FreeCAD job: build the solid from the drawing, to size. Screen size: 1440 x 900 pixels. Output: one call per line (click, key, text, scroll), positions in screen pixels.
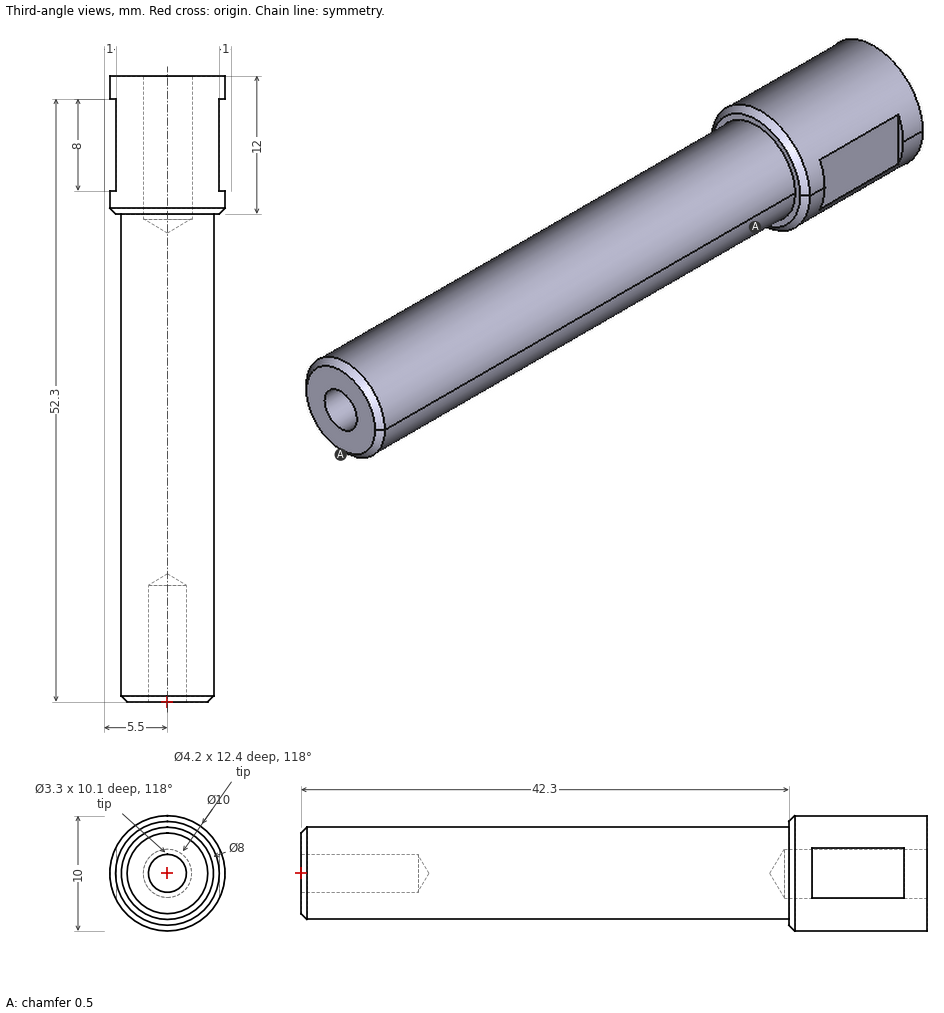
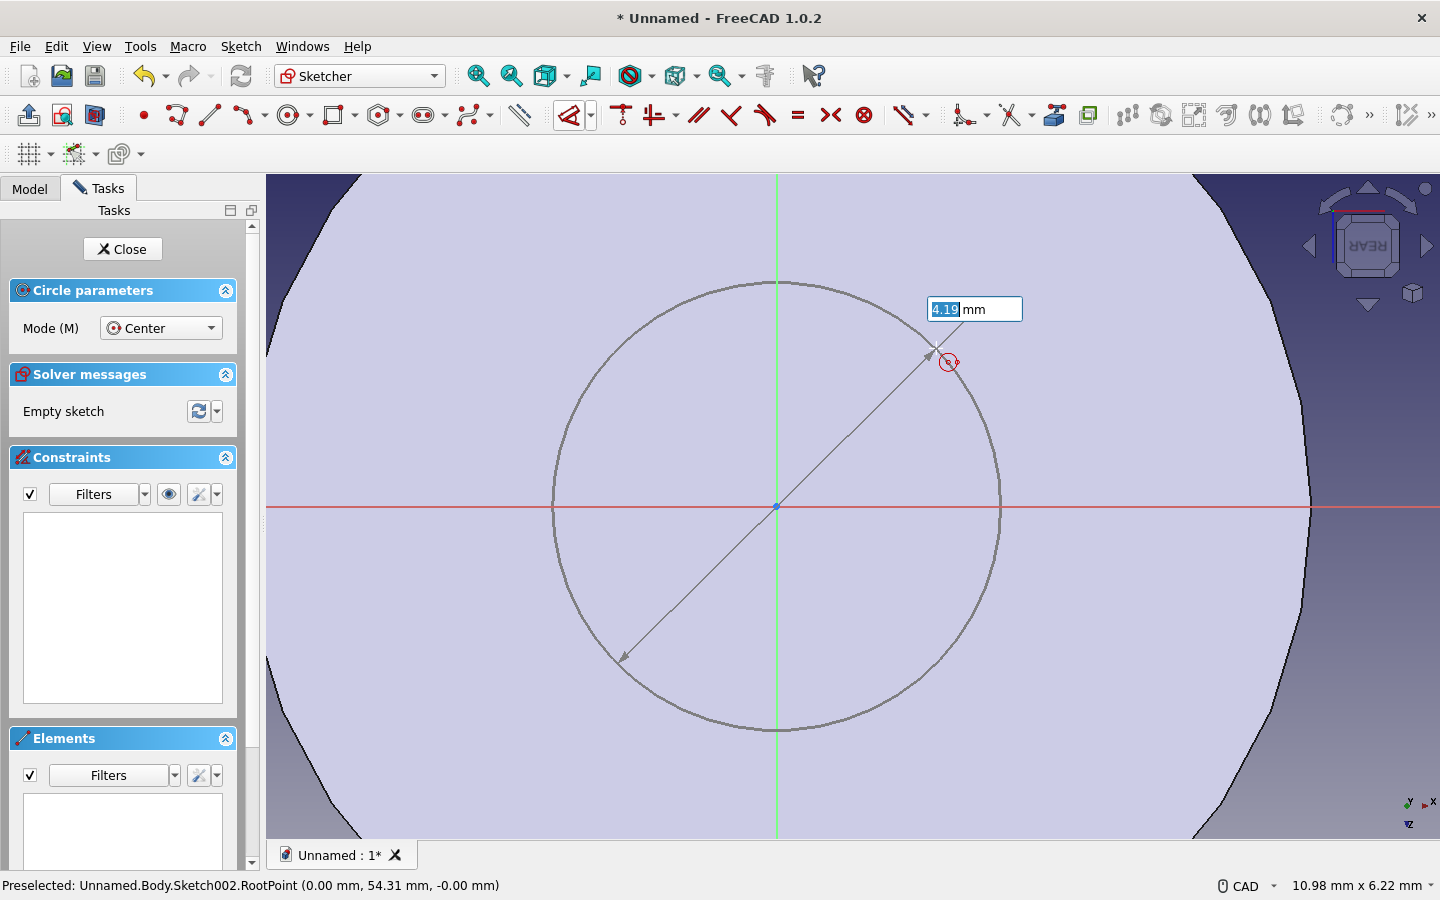
text(4.2)
key(Return)
key(Escape)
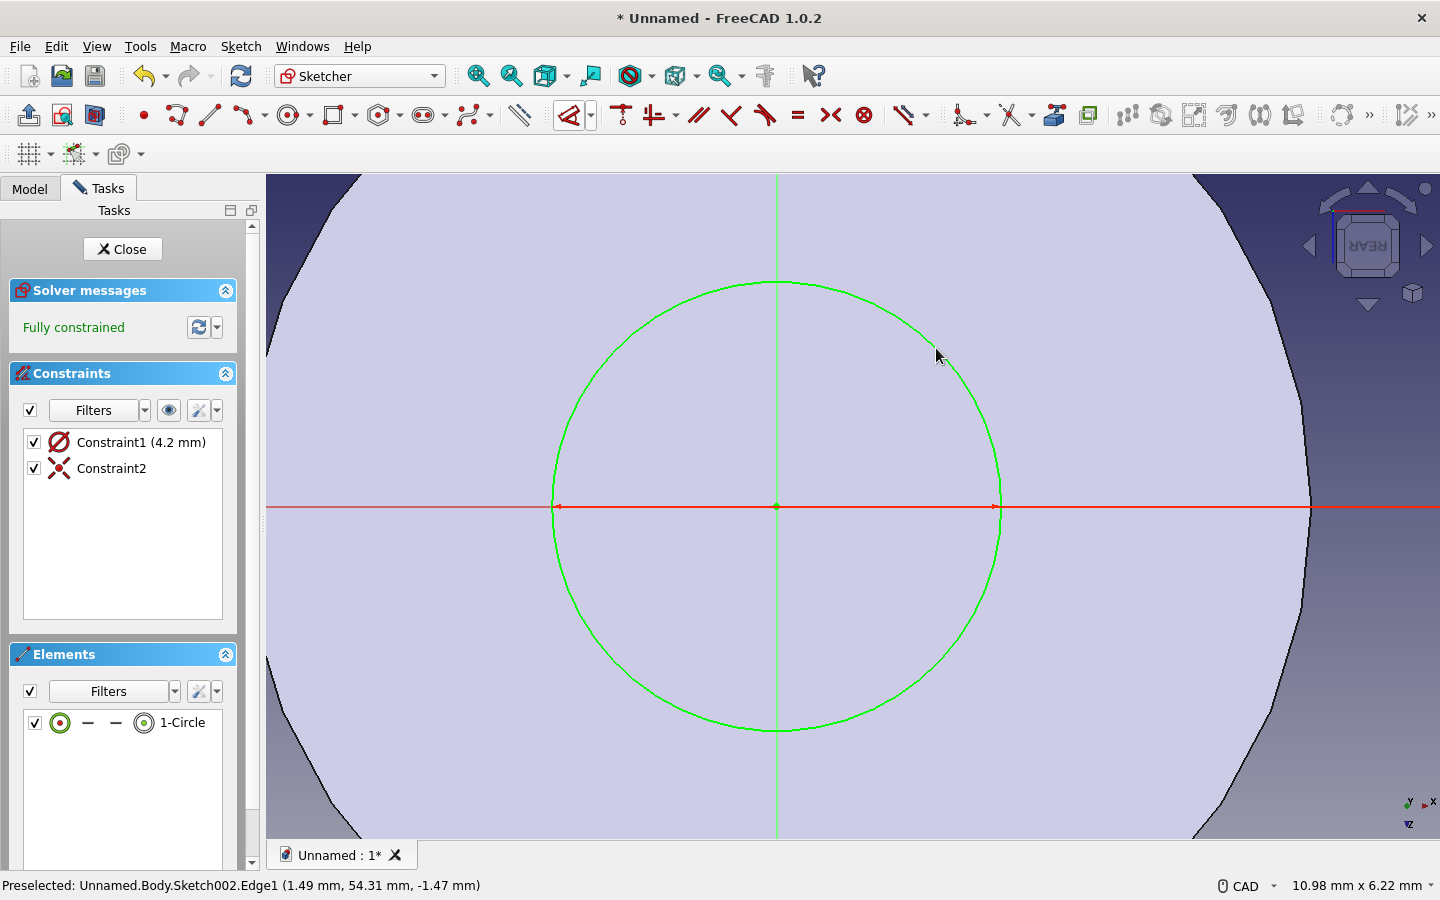
click(123, 249)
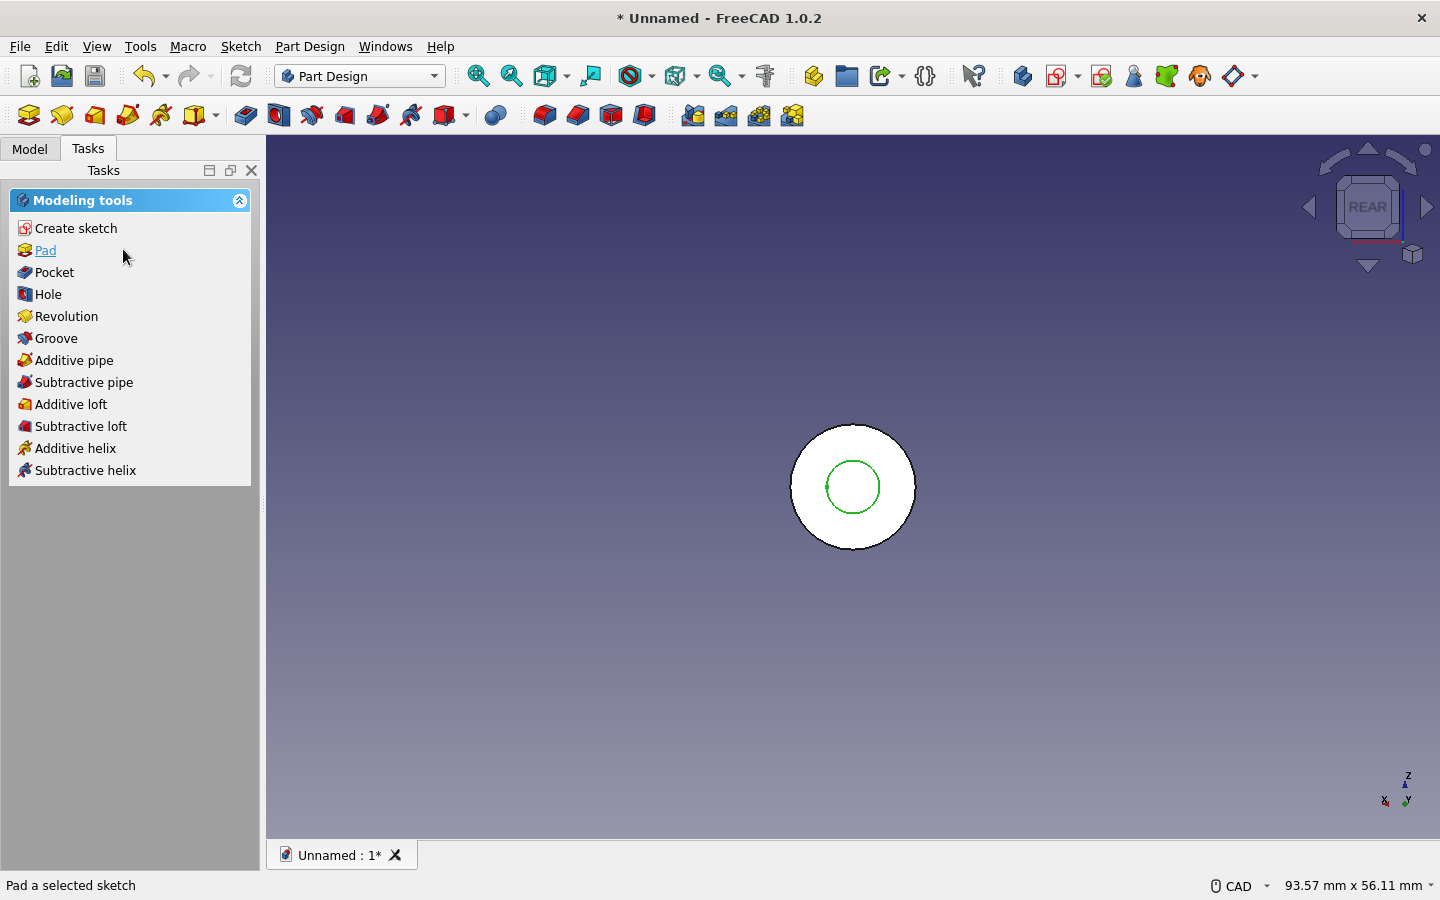
click(279, 116)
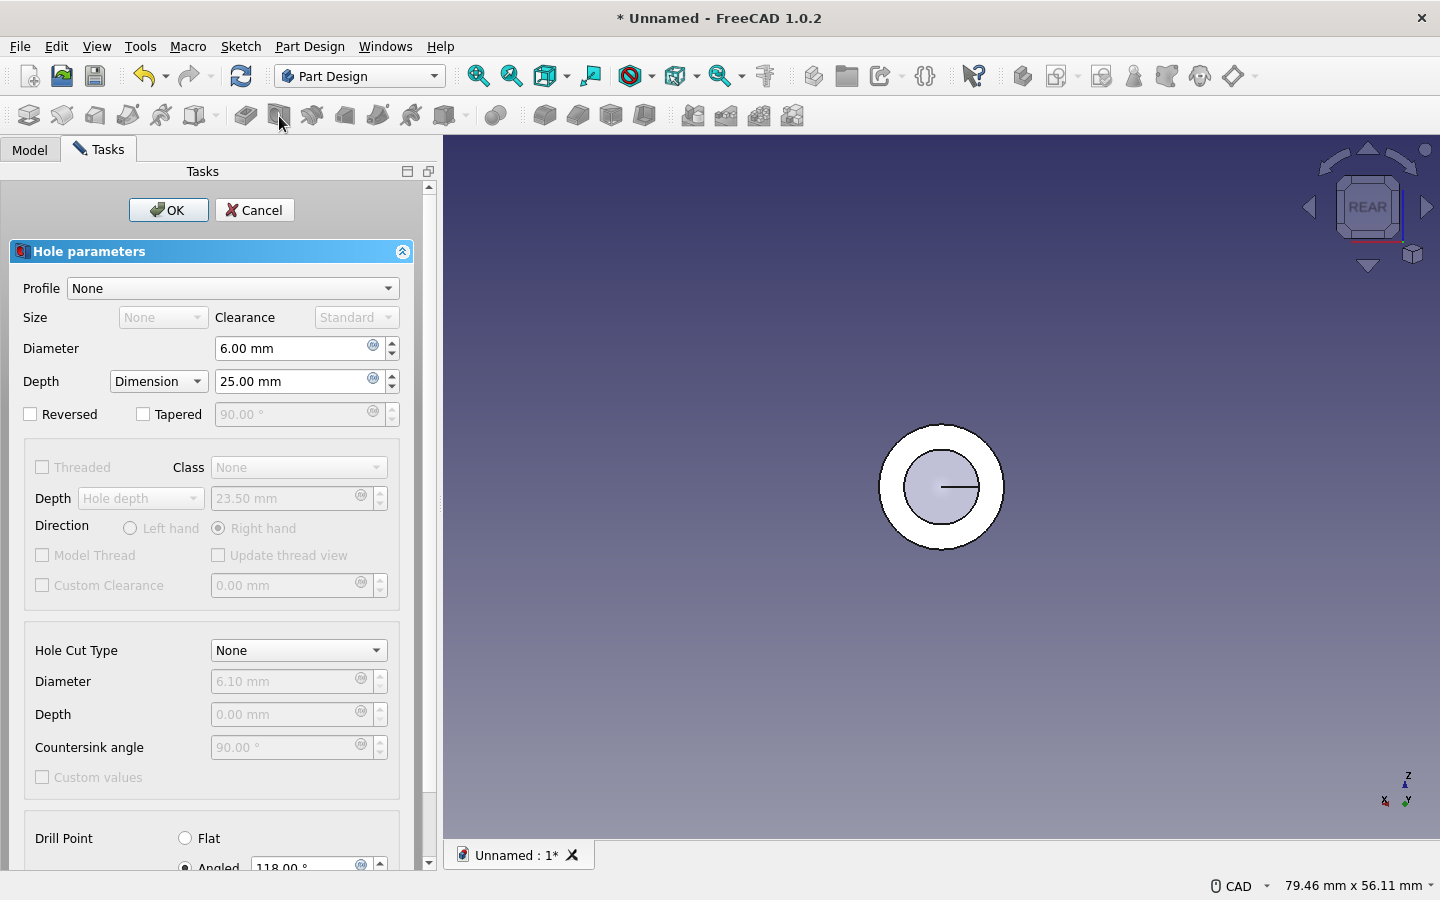
triple_click(300, 348)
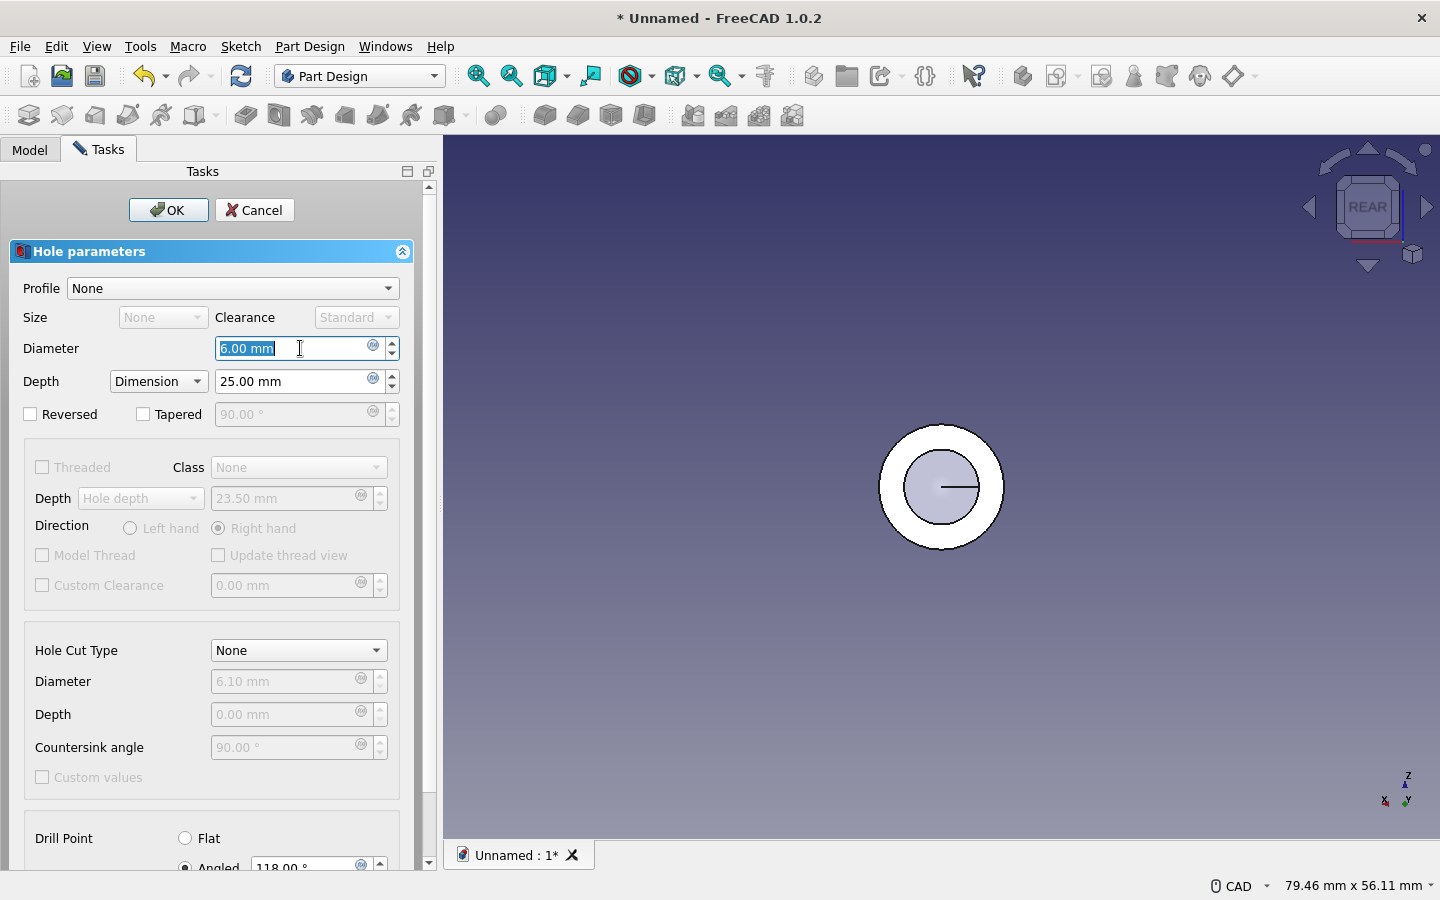
text(4.2)
key(Tab)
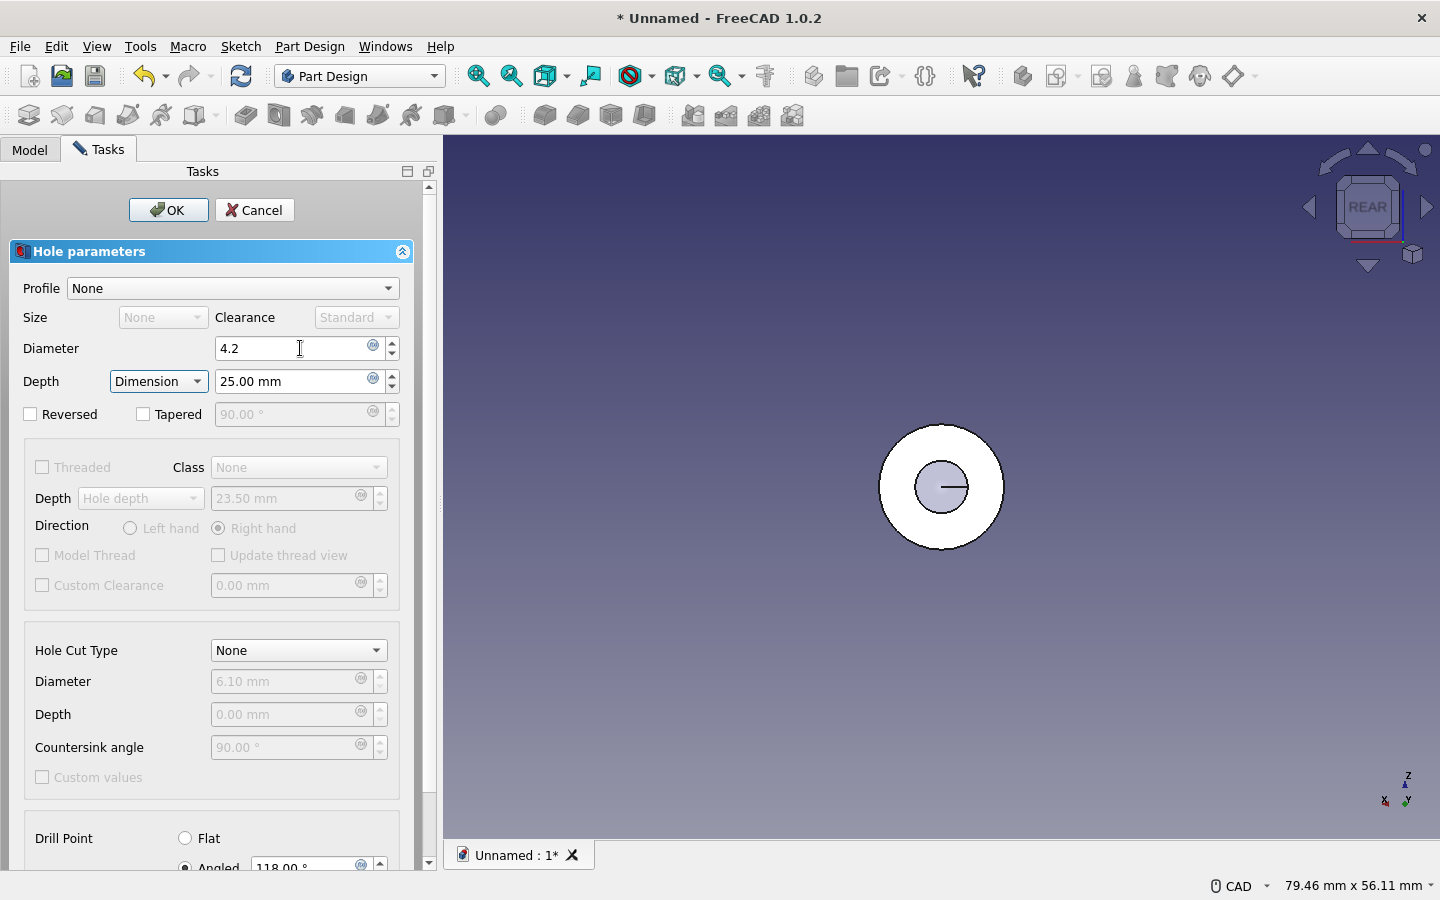
triple_click(300, 382)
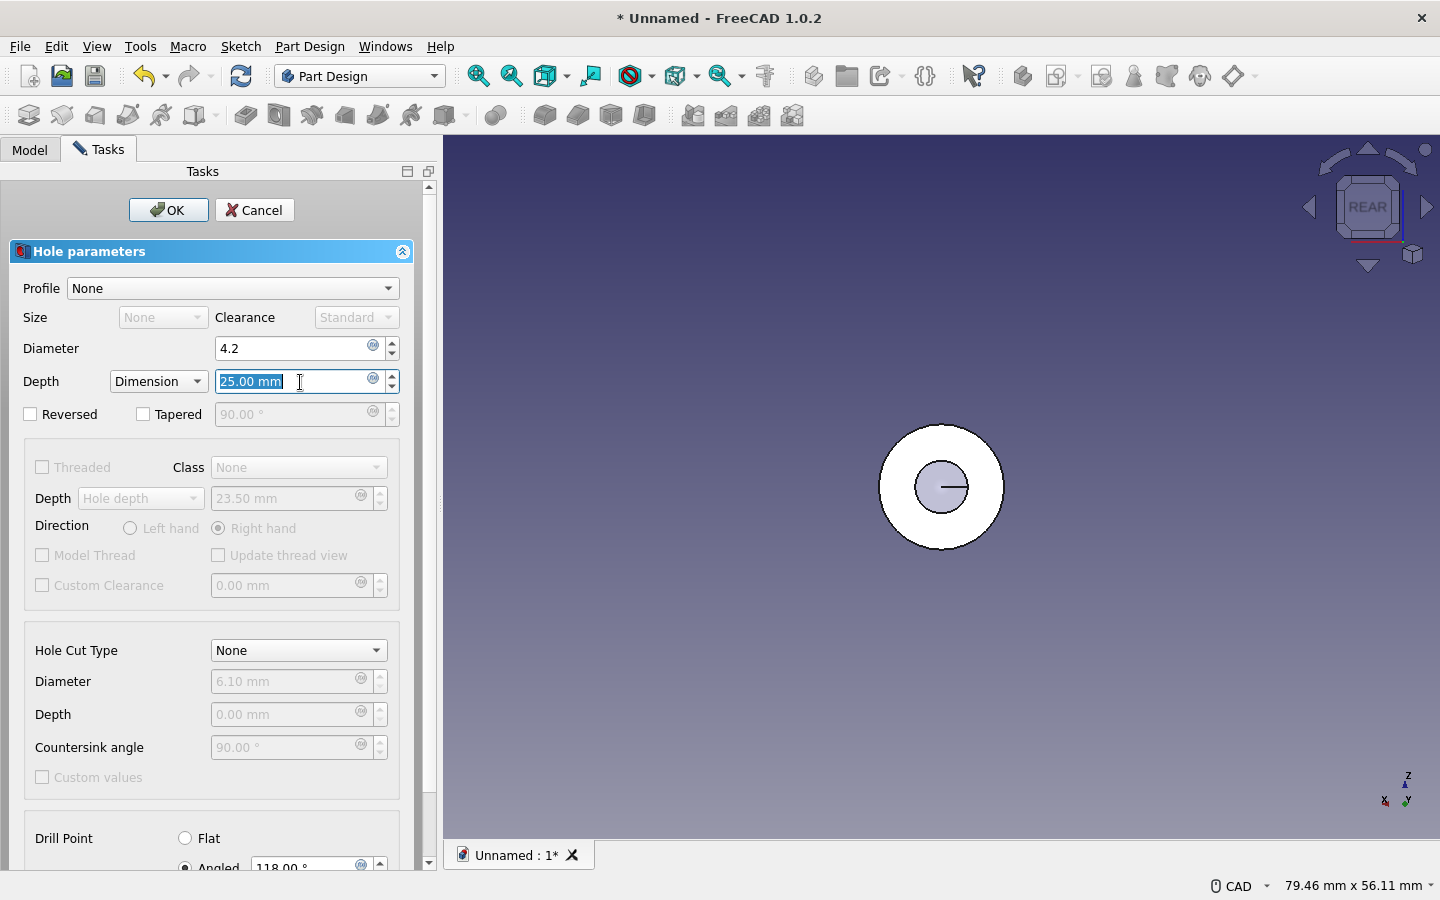
text(12.4)
key(Tab)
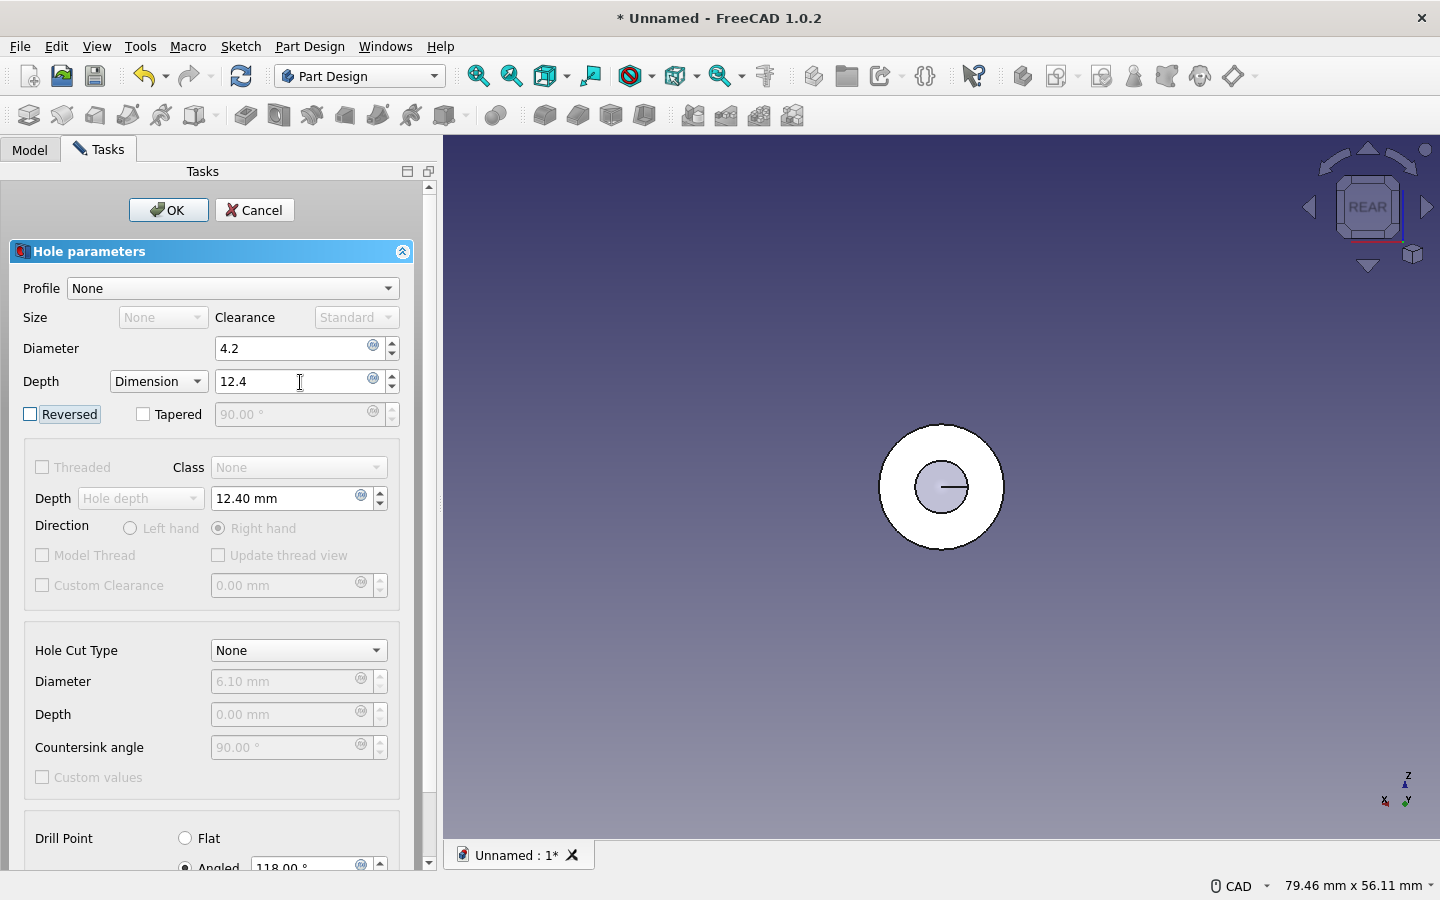
click(169, 210)